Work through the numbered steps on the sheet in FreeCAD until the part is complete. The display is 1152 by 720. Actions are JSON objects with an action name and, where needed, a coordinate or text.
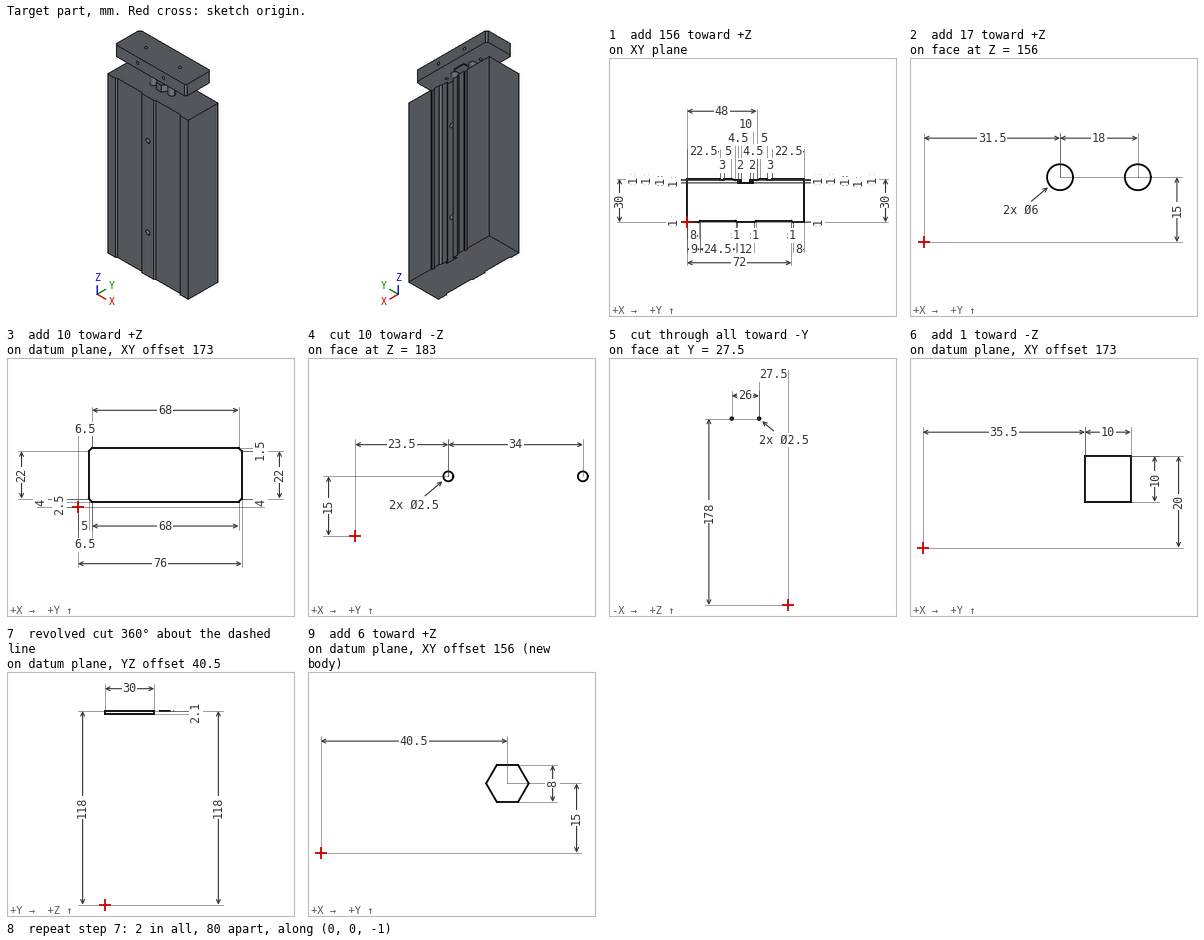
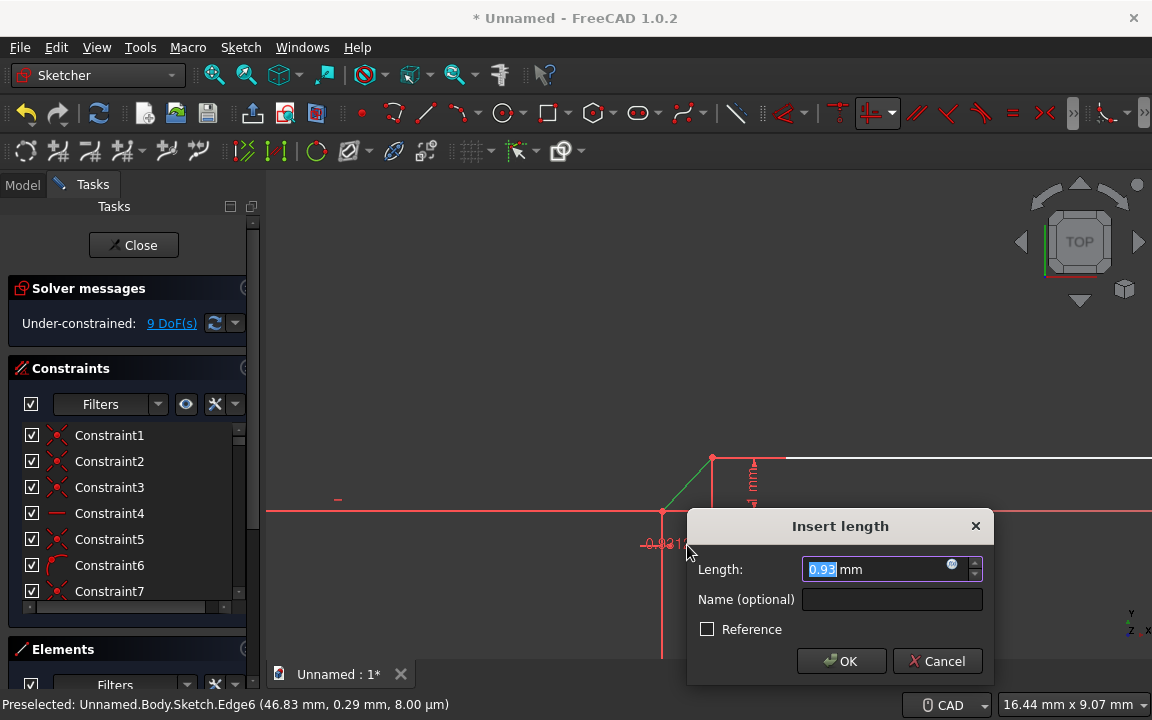
{"action": "type", "text": "1"}
{"action": "key", "text": "Return"}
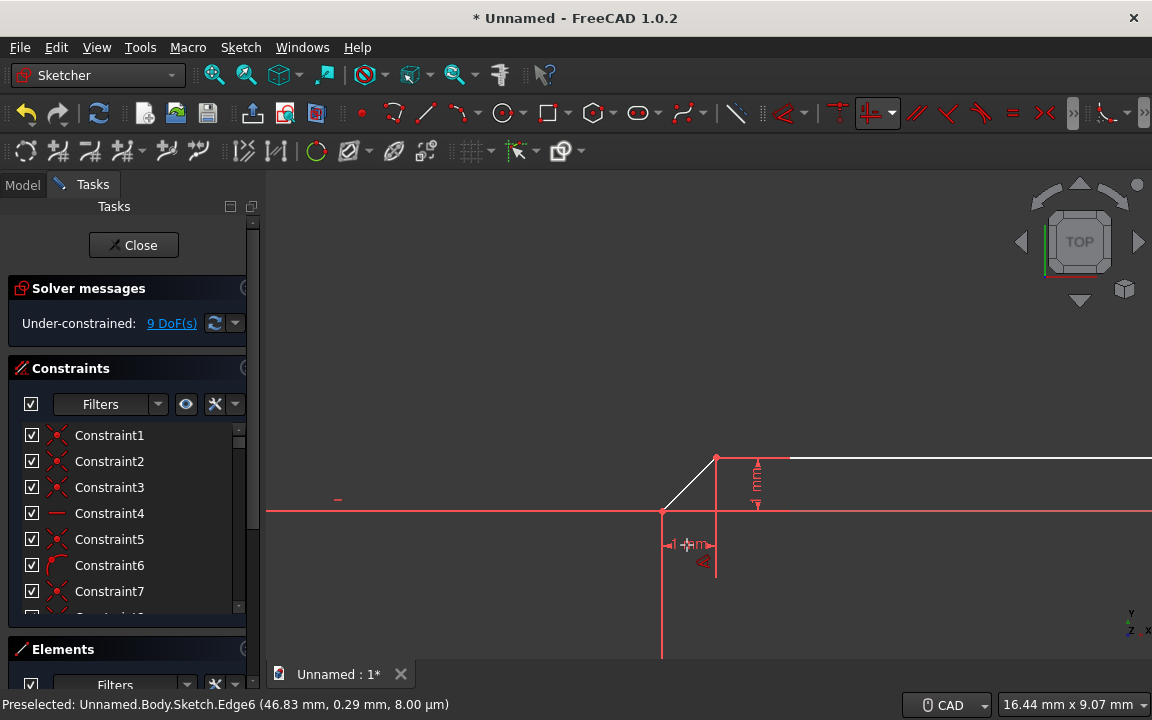
{"action": "scroll", "coordinate": [679, 503], "scroll_direction": "down", "scroll_amount": 11}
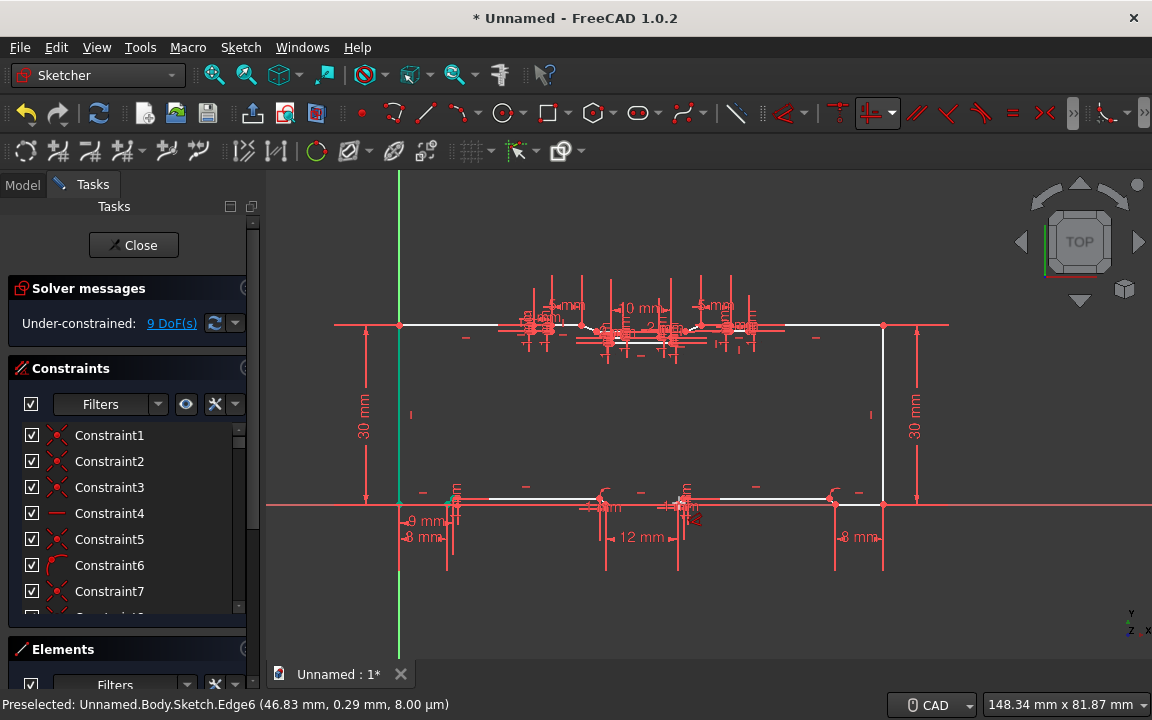
{"action": "scroll", "coordinate": [831, 500], "scroll_direction": "up", "scroll_amount": 10}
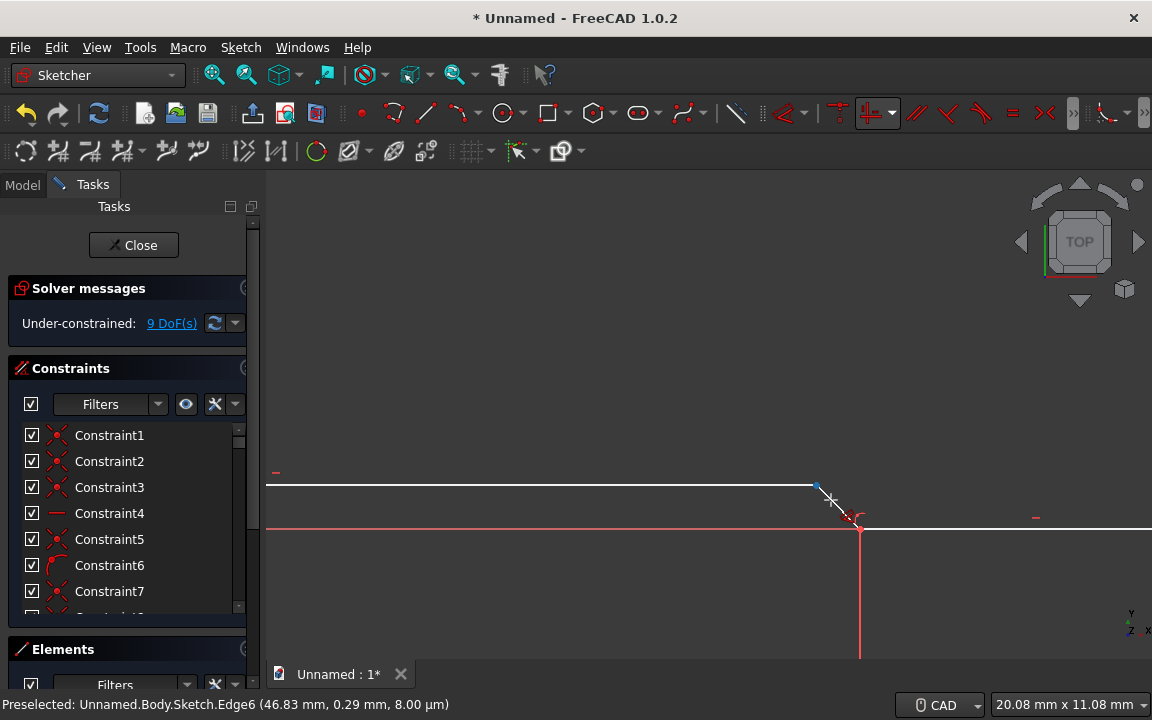
{"action": "left_click", "coordinate": [830, 498]}
{"action": "left_click", "coordinate": [838, 563]}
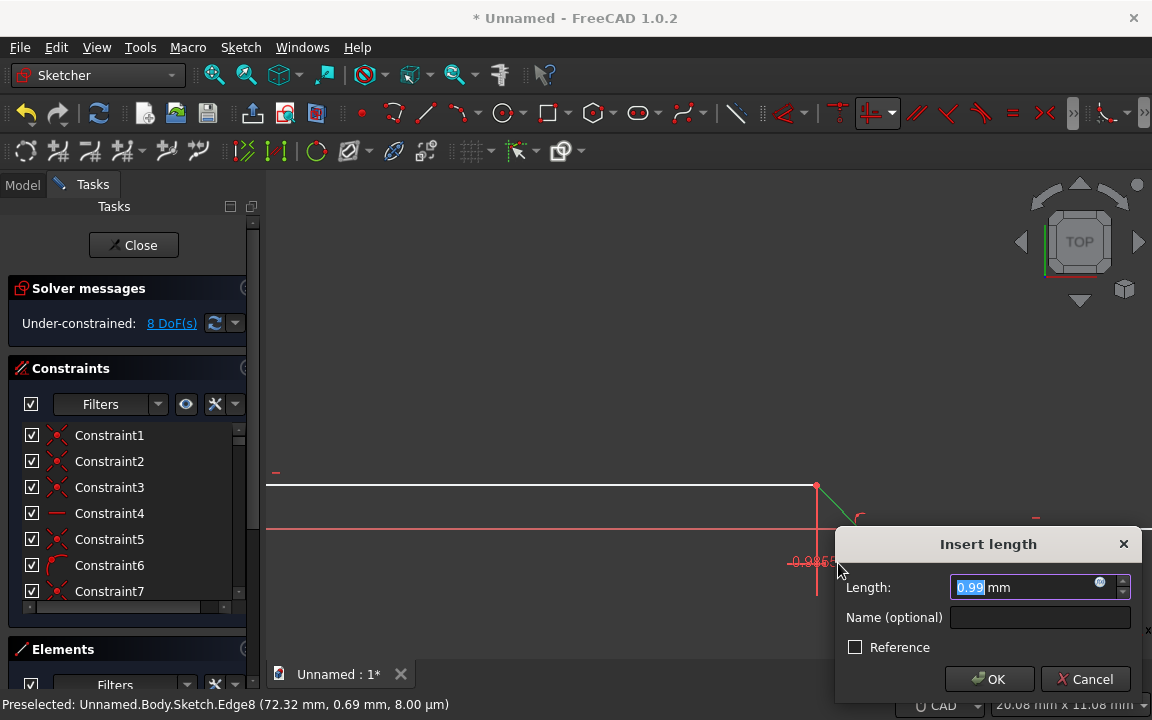
{"action": "type", "text": "1"}
{"action": "key", "text": "Return"}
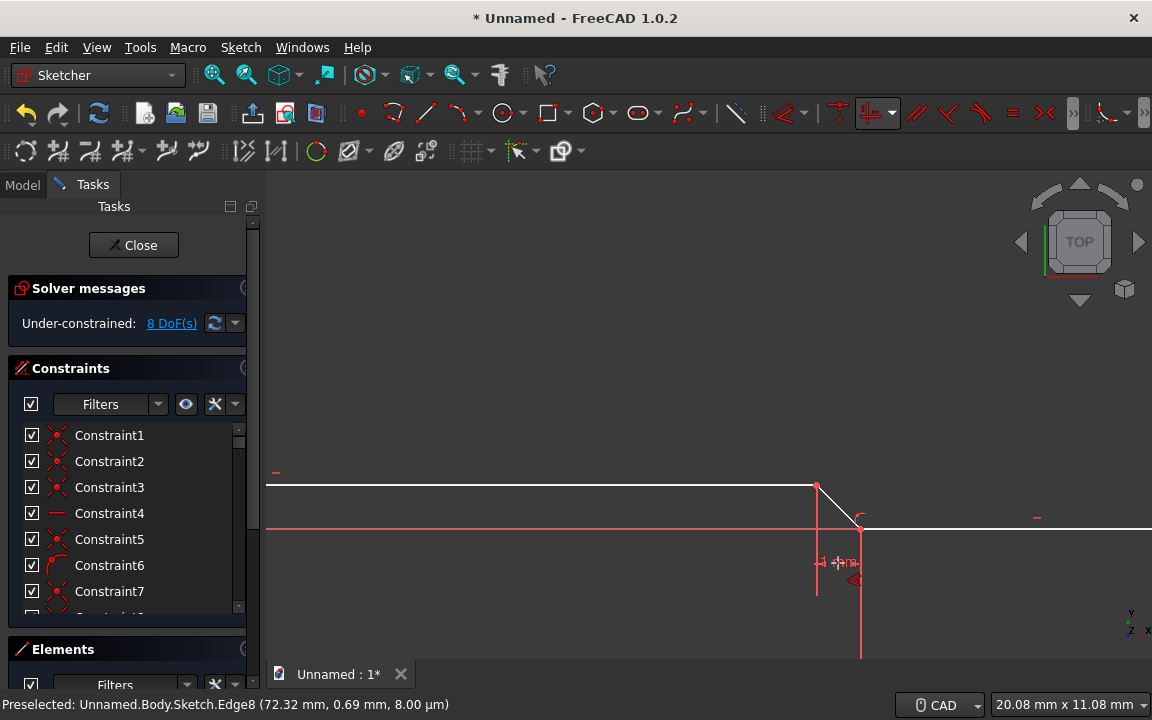
{"action": "scroll", "coordinate": [831, 500], "scroll_direction": "down", "scroll_amount": 10}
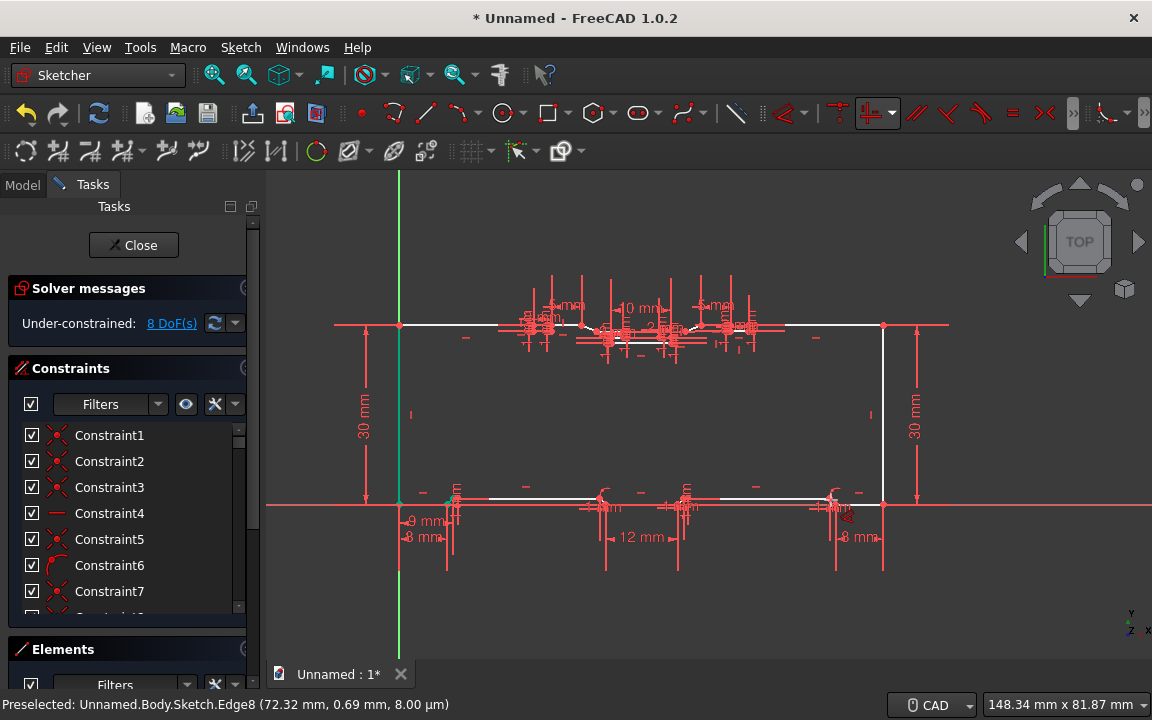
{"action": "scroll", "coordinate": [697, 327], "scroll_direction": "up", "scroll_amount": 10}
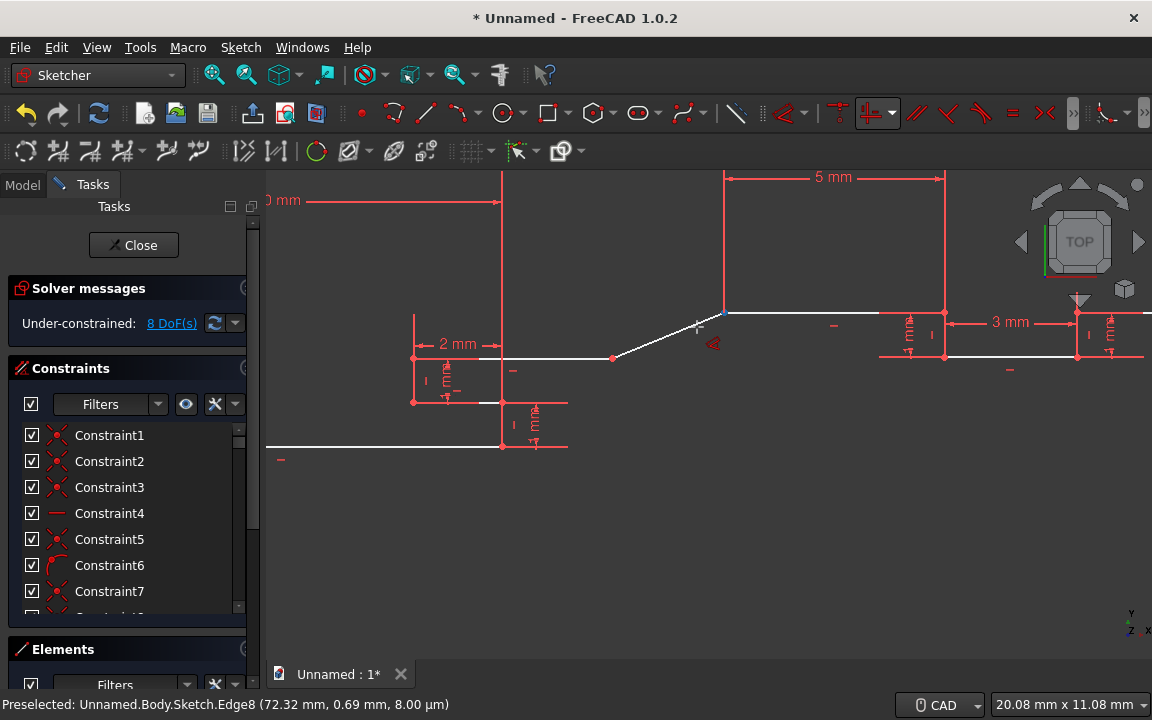
{"action": "left_click", "coordinate": [691, 327]}
{"action": "left_click", "coordinate": [758, 336]}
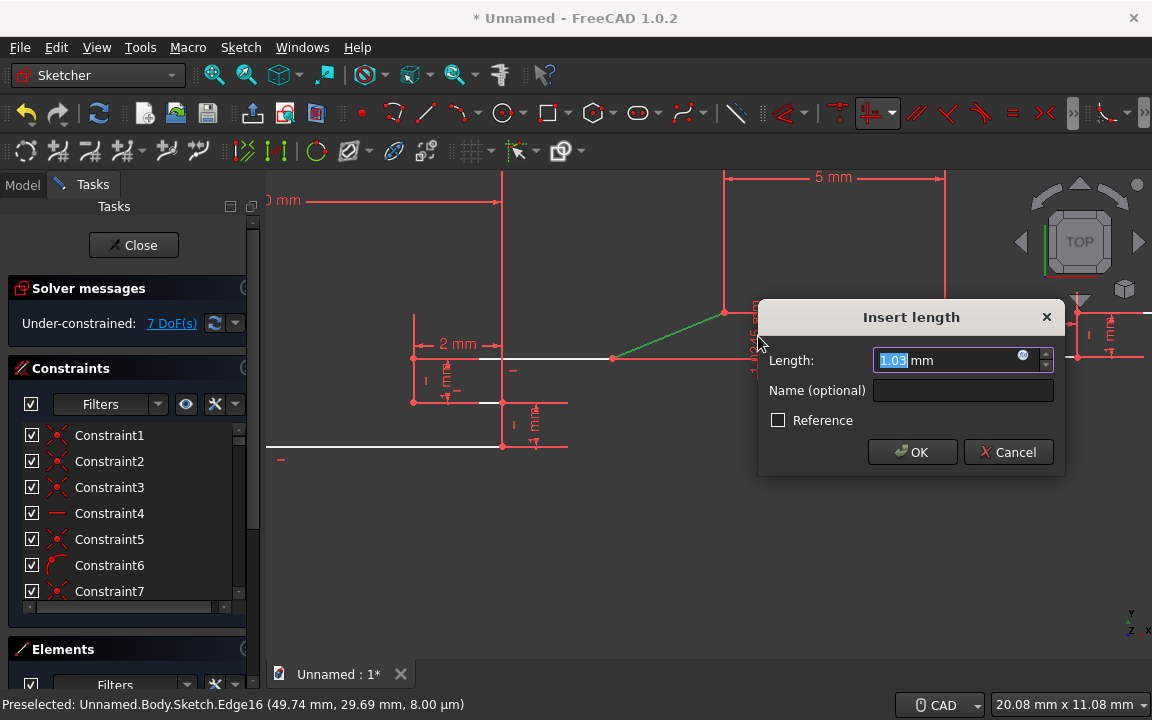
{"action": "type", "text": "1"}
{"action": "key", "text": "Return"}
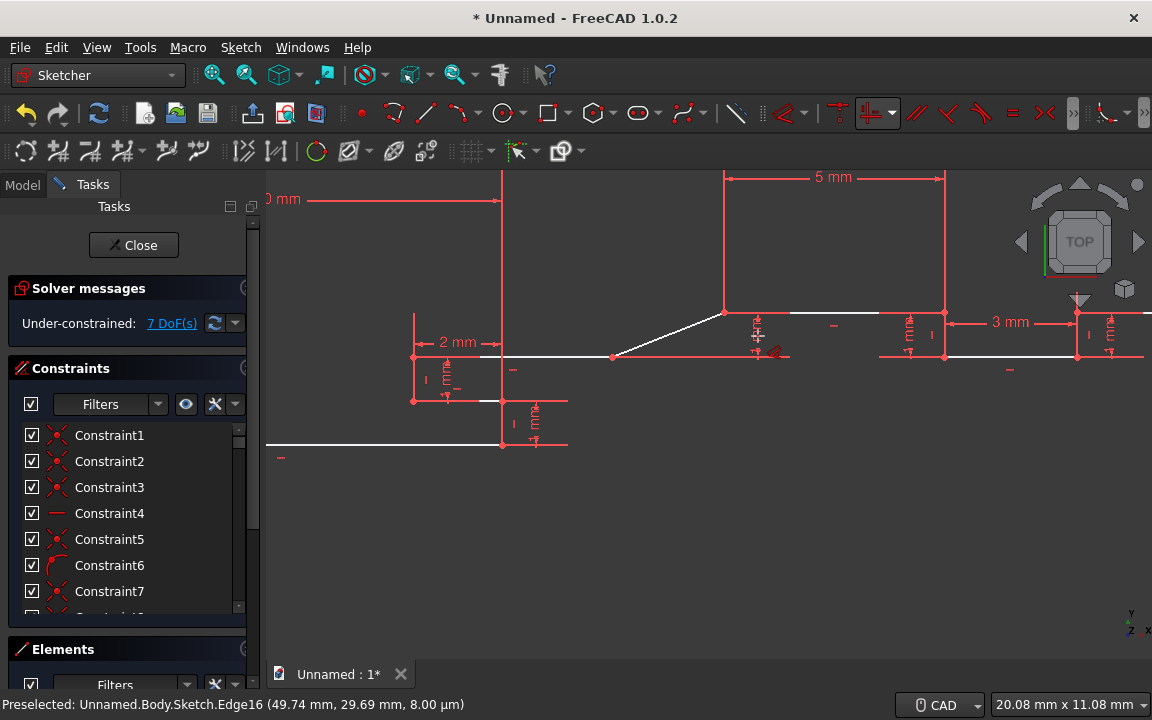
{"action": "scroll", "coordinate": [696, 327], "scroll_direction": "down", "scroll_amount": 10}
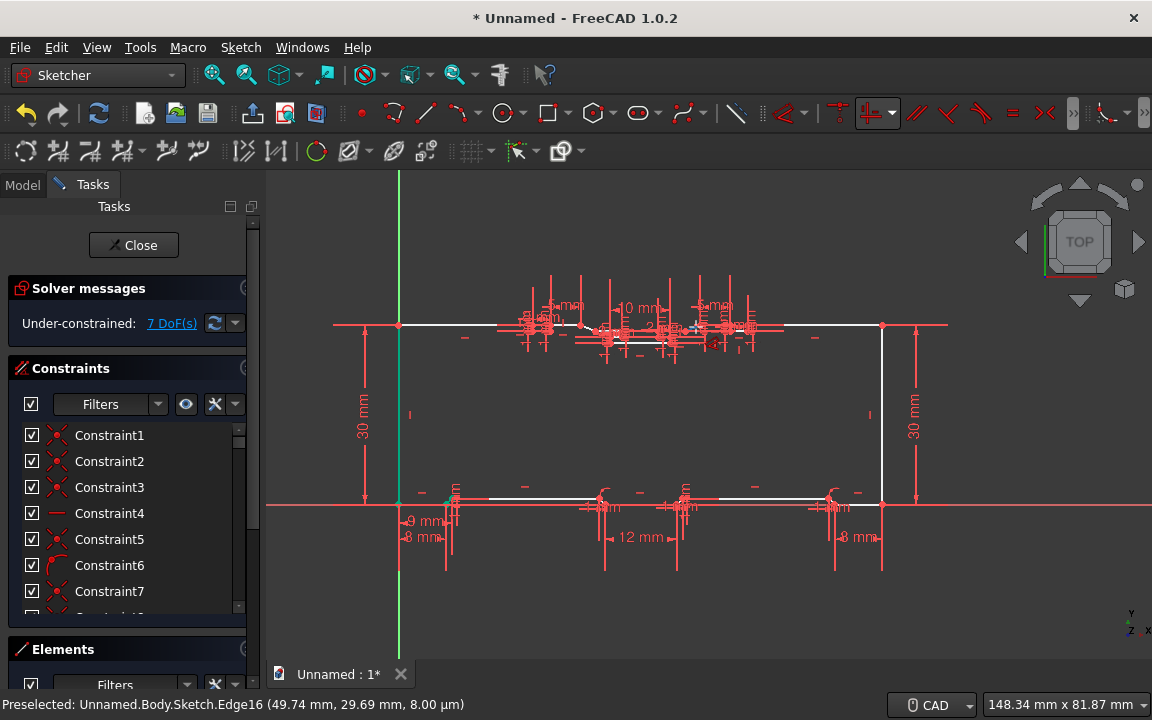
{"action": "scroll", "coordinate": [677, 331], "scroll_direction": "up", "scroll_amount": 3}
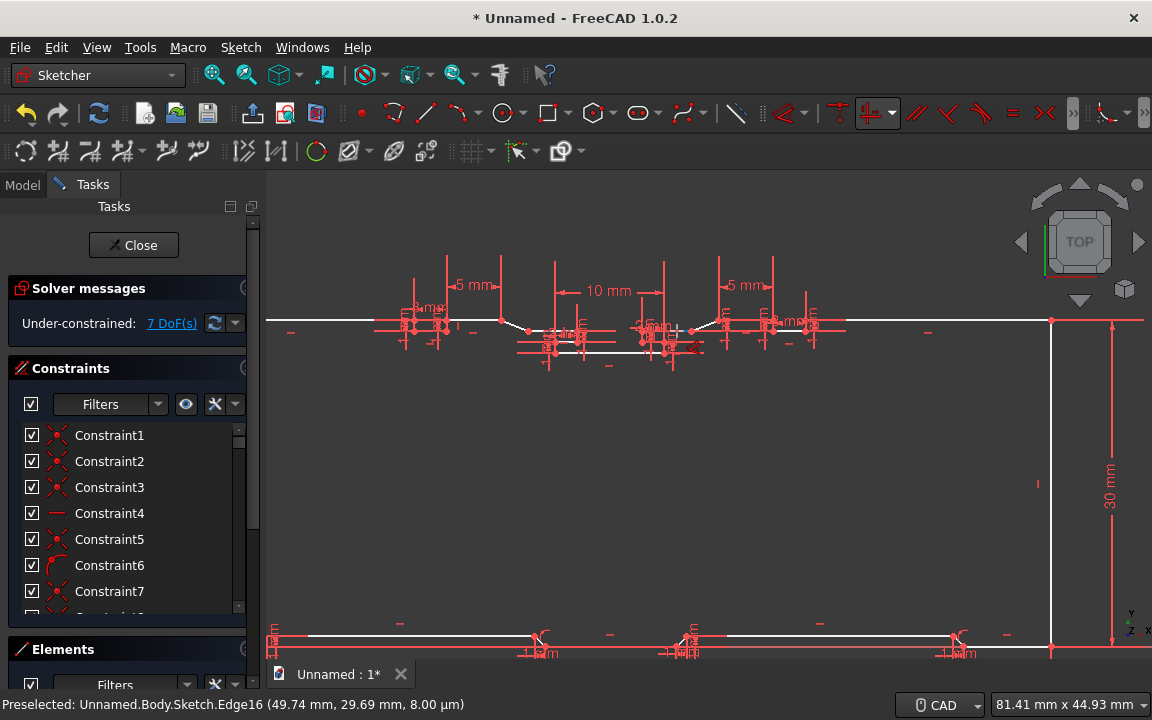
{"action": "left_click", "coordinate": [677, 331]}
{"action": "left_click", "coordinate": [667, 389]}